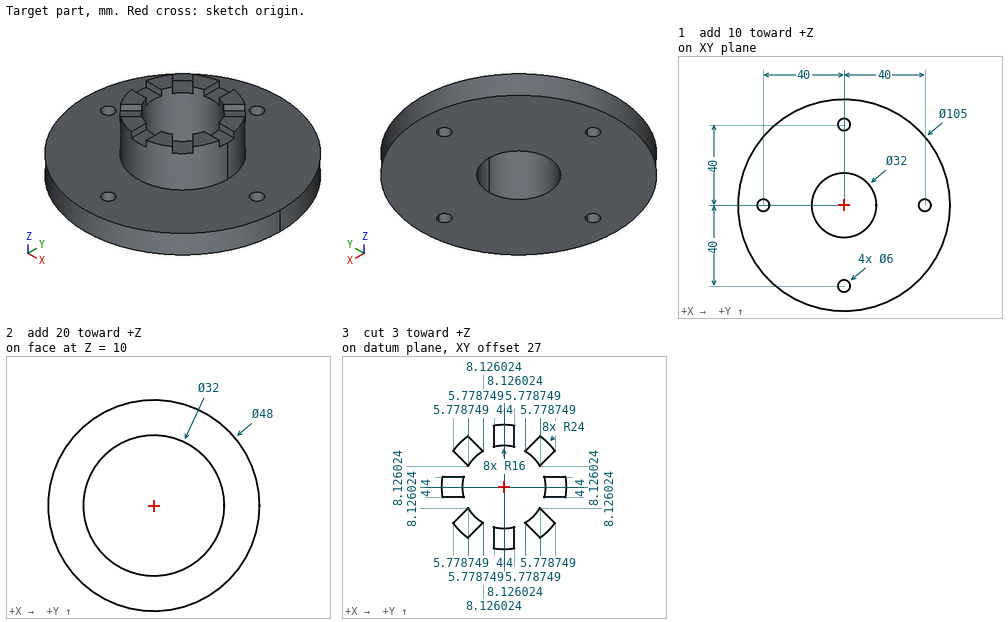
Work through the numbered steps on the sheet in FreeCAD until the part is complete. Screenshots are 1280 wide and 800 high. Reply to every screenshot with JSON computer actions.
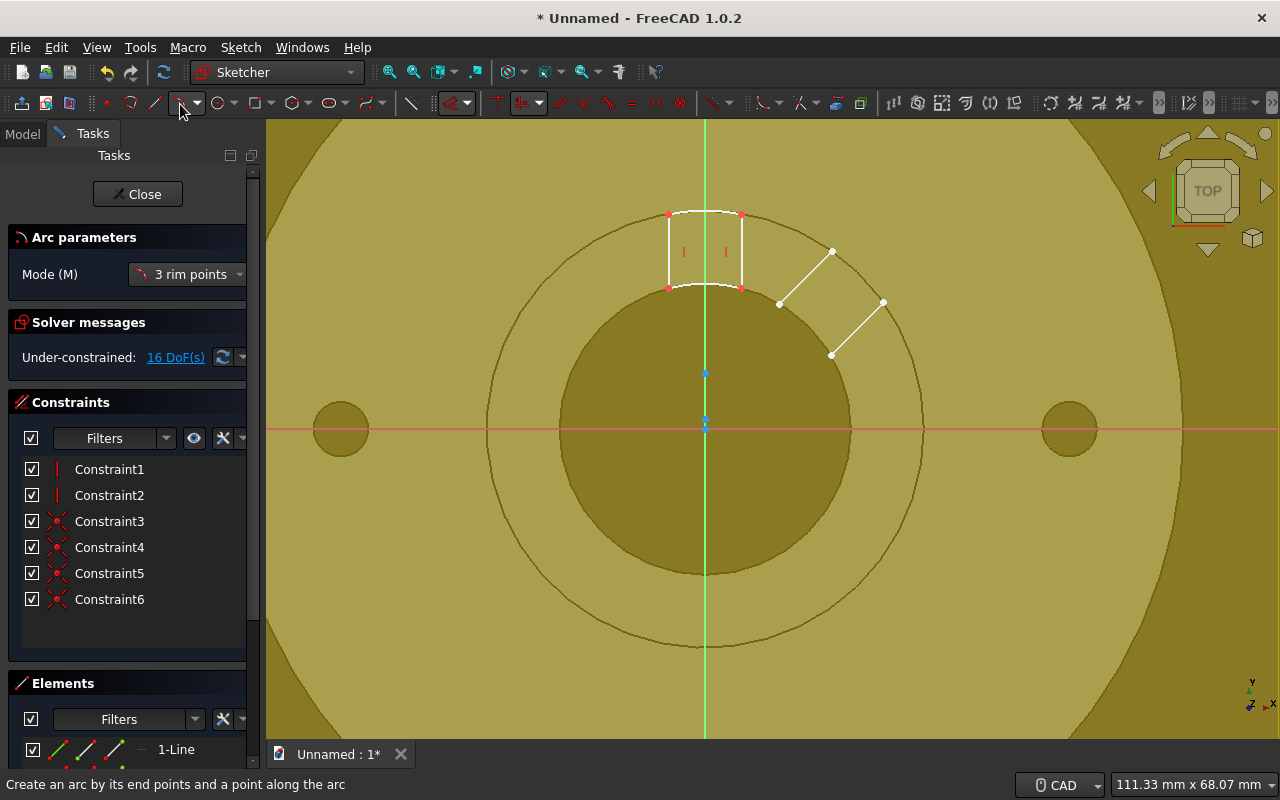
{"action": "left_click", "coordinate": [779, 305]}
{"action": "left_click", "coordinate": [831, 356]}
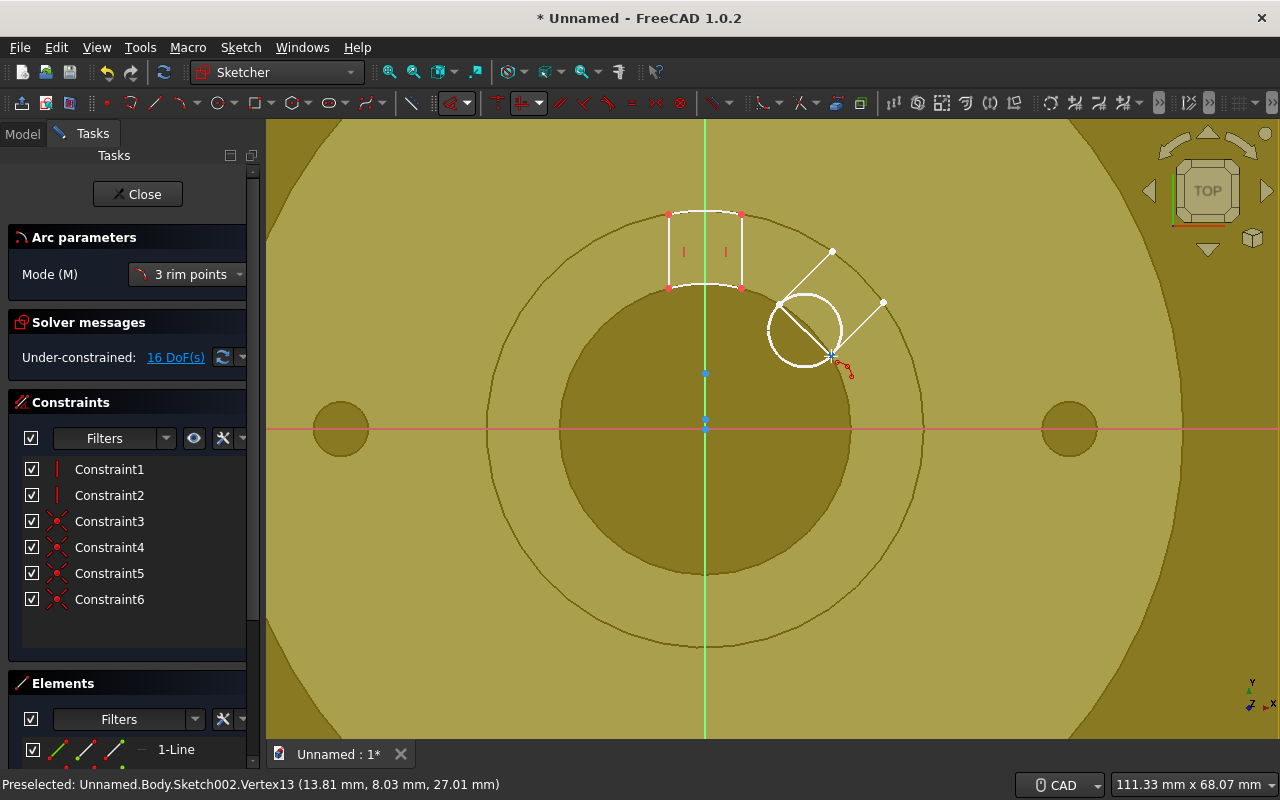
{"action": "scroll", "coordinate": [808, 326], "scroll_direction": "up", "scroll_amount": 7}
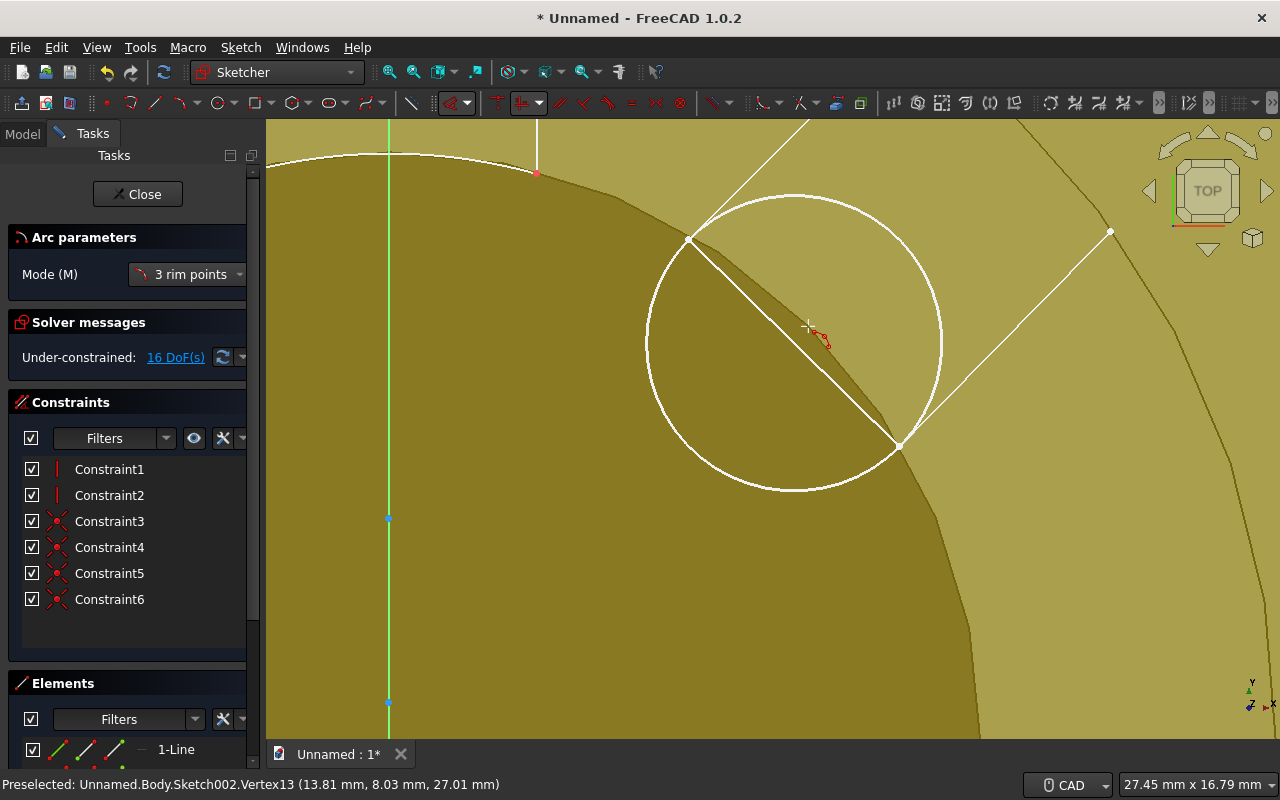
{"action": "left_click", "coordinate": [807, 325]}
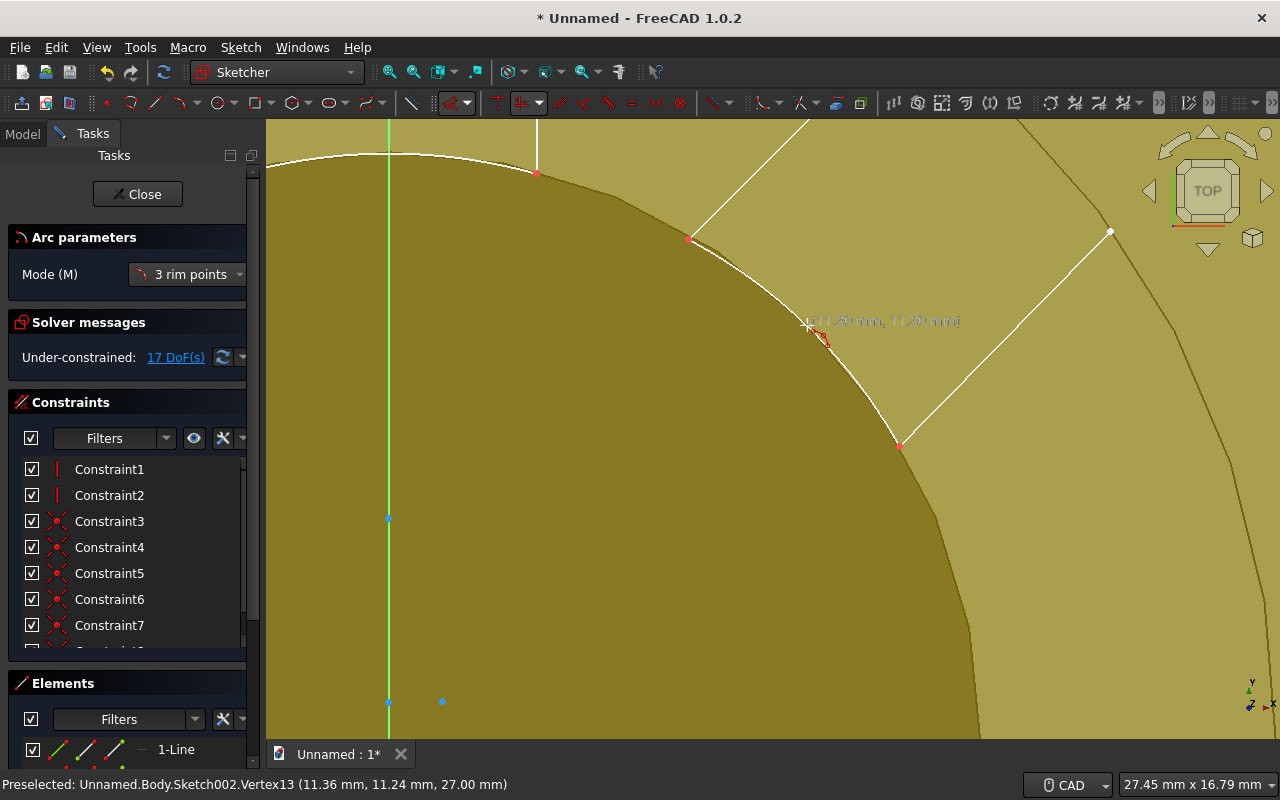
{"action": "scroll", "coordinate": [808, 326], "scroll_direction": "down", "scroll_amount": 7}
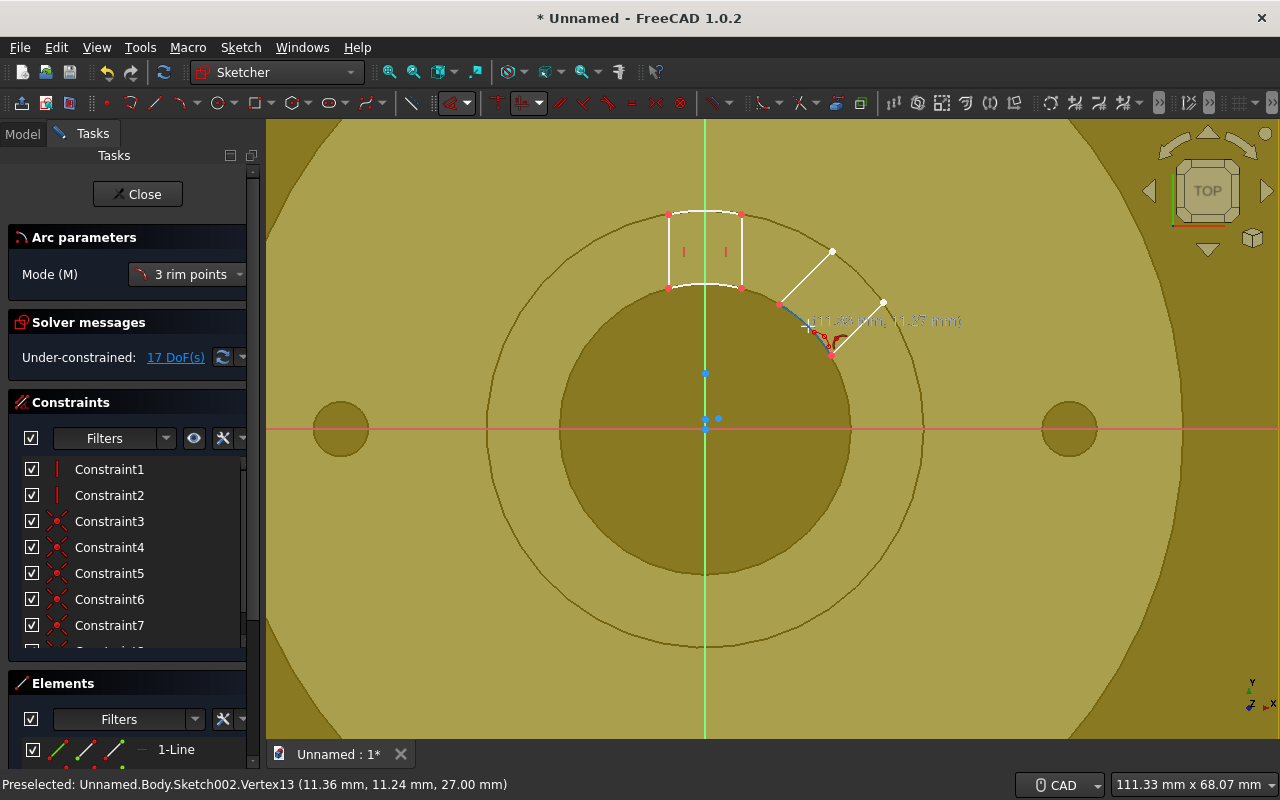
{"action": "left_click", "coordinate": [883, 303]}
{"action": "left_click", "coordinate": [832, 252]}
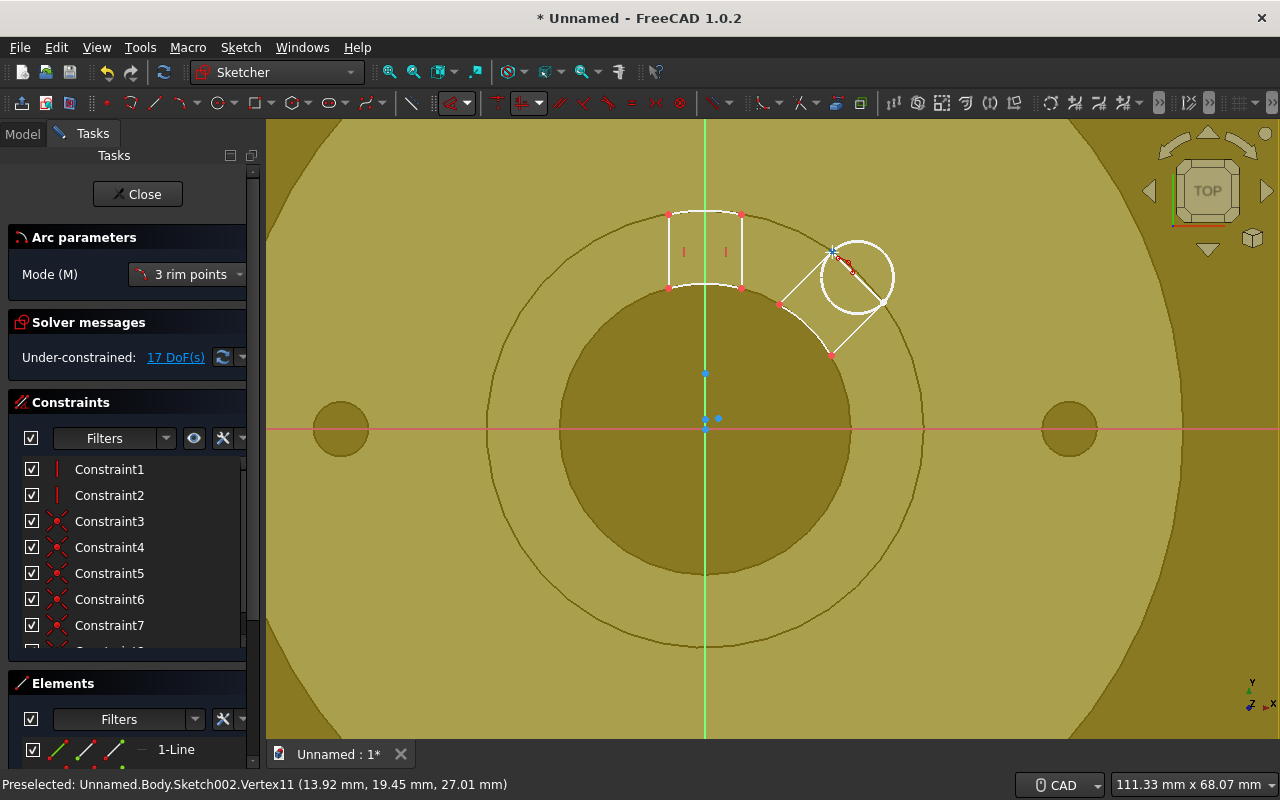
{"action": "scroll", "coordinate": [860, 275], "scroll_direction": "up", "scroll_amount": 9}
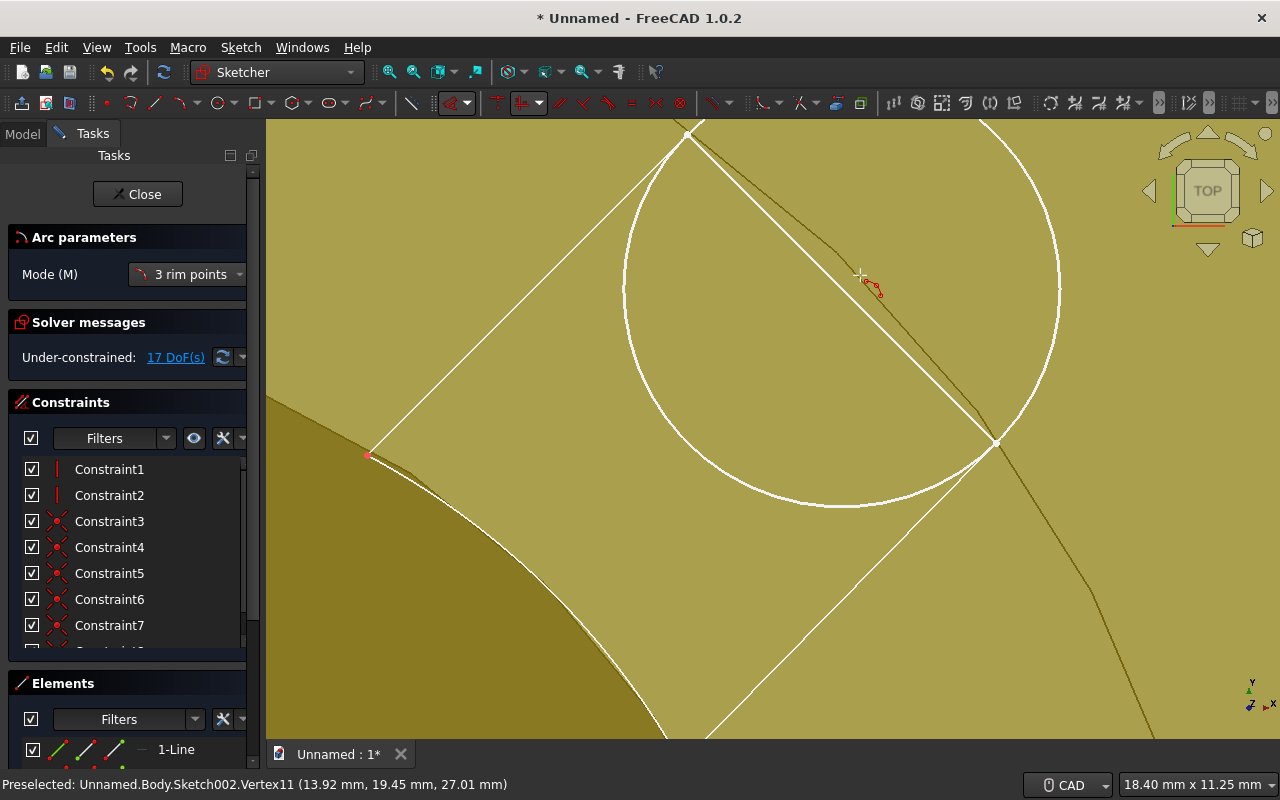
{"action": "left_click", "coordinate": [856, 271]}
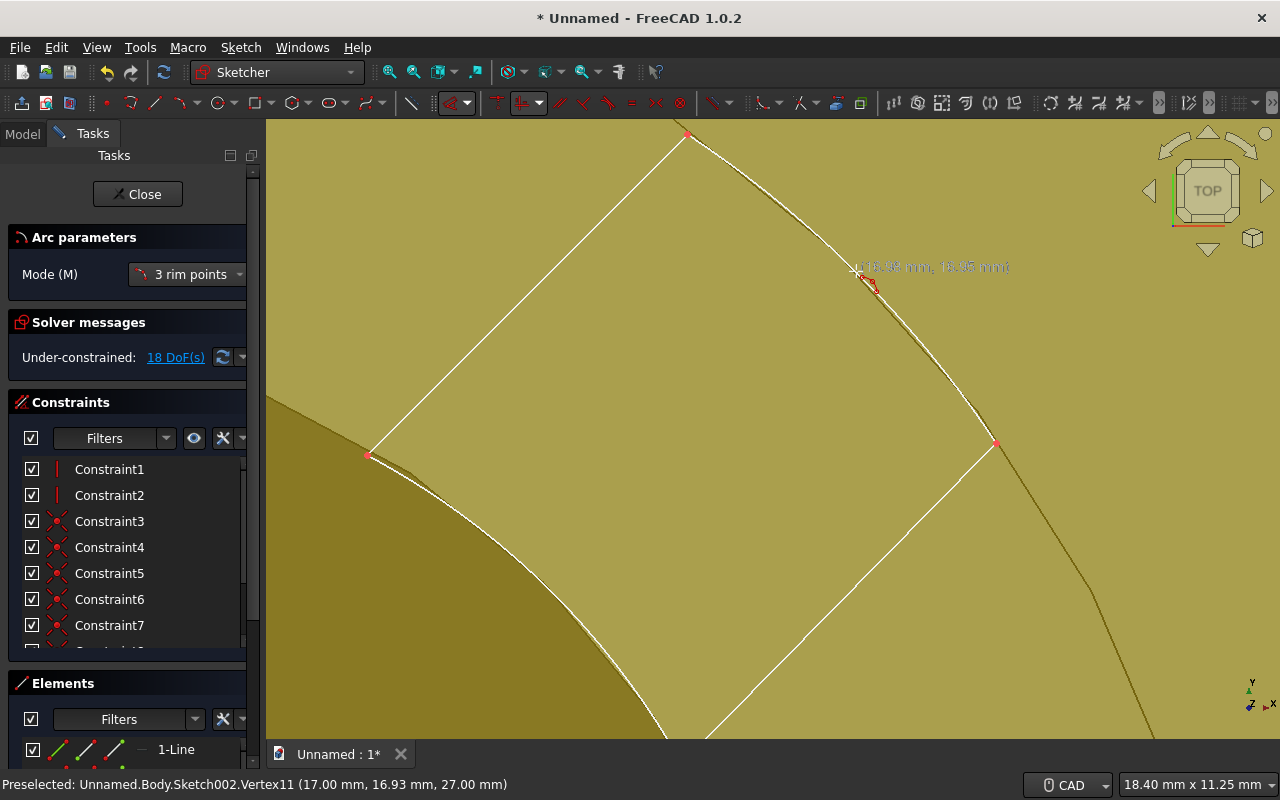
{"action": "left_click", "coordinate": [156, 104]}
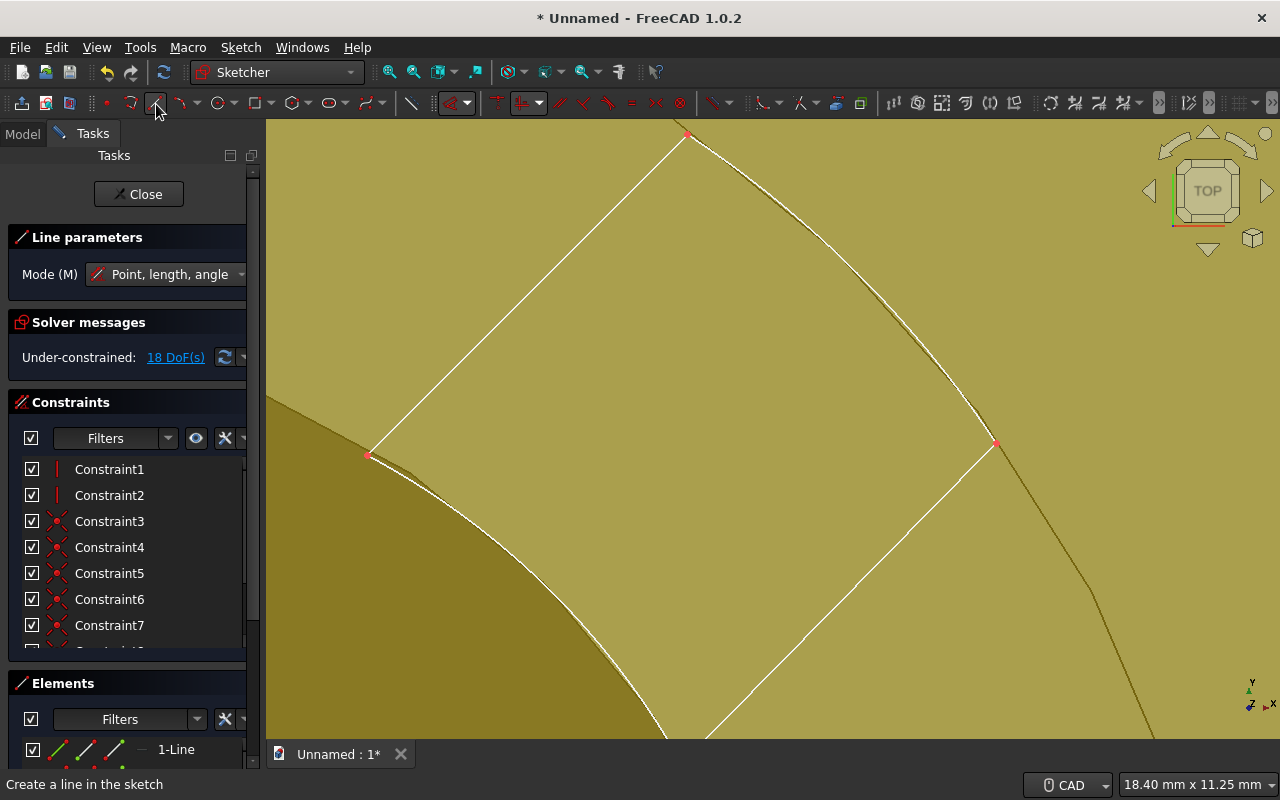
{"action": "scroll", "coordinate": [860, 275], "scroll_direction": "down", "scroll_amount": 9}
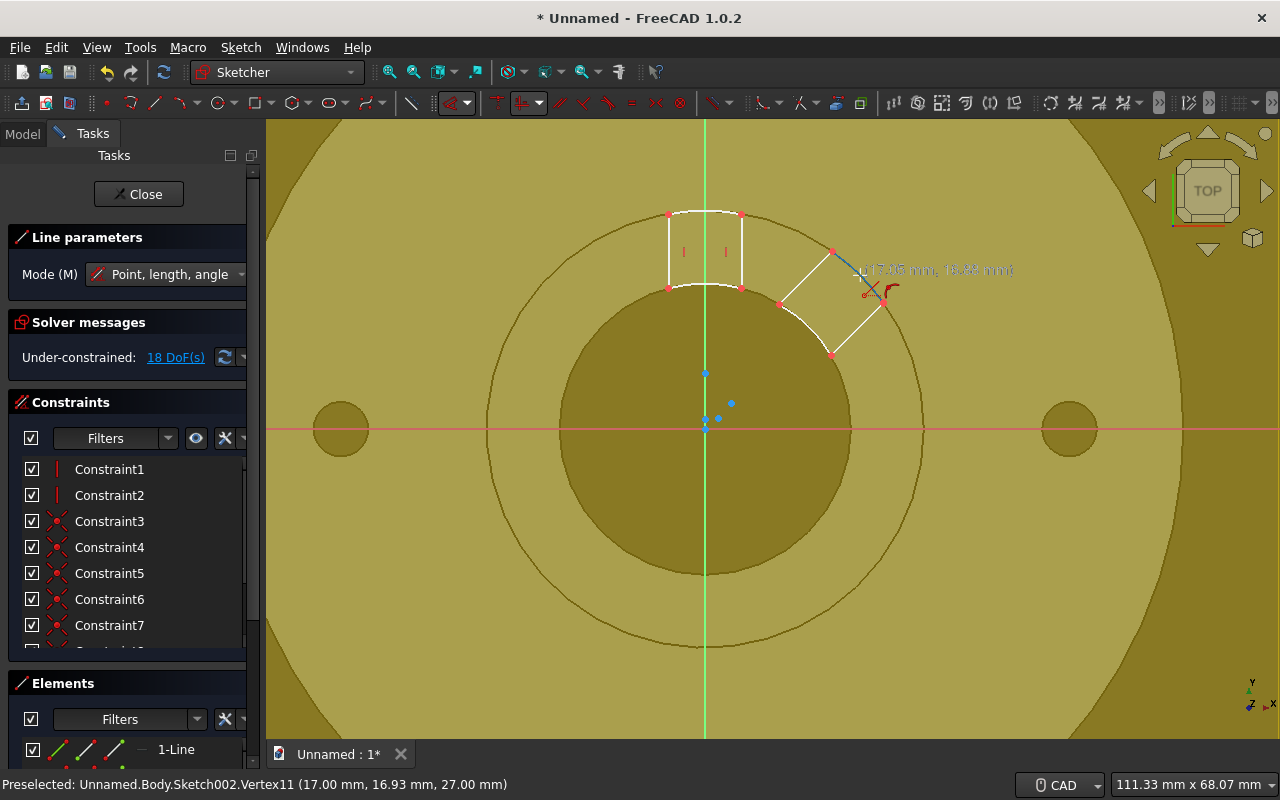
{"action": "left_click", "coordinate": [921, 393]}
{"action": "left_click", "coordinate": [846, 393]}